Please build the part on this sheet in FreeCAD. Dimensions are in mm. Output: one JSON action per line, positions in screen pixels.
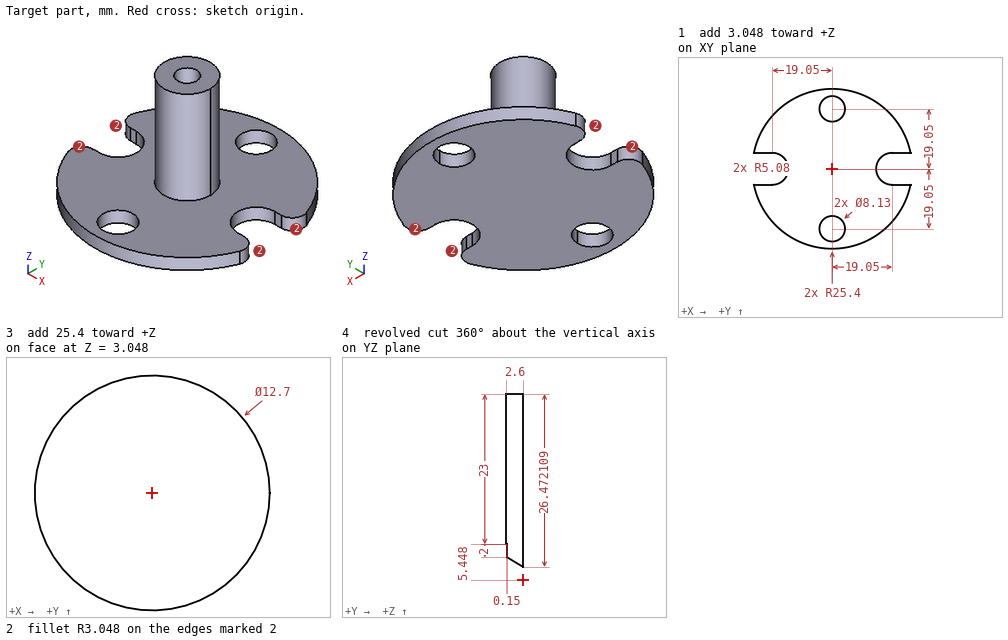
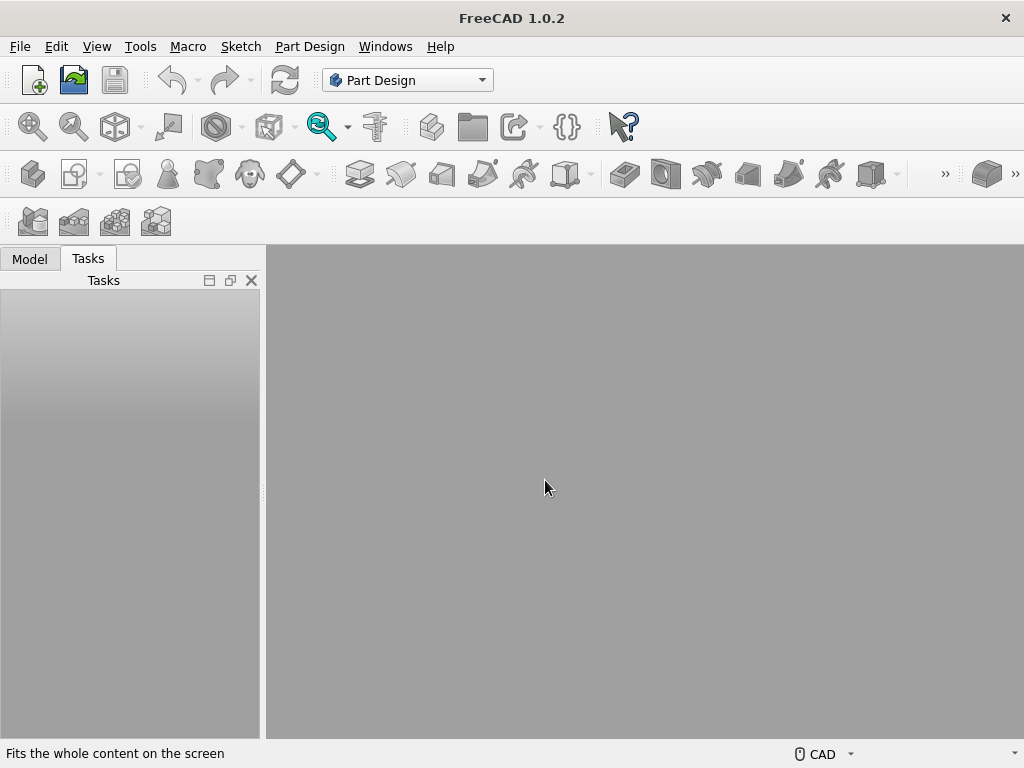
{"action": "left_click", "coordinate": [33, 80]}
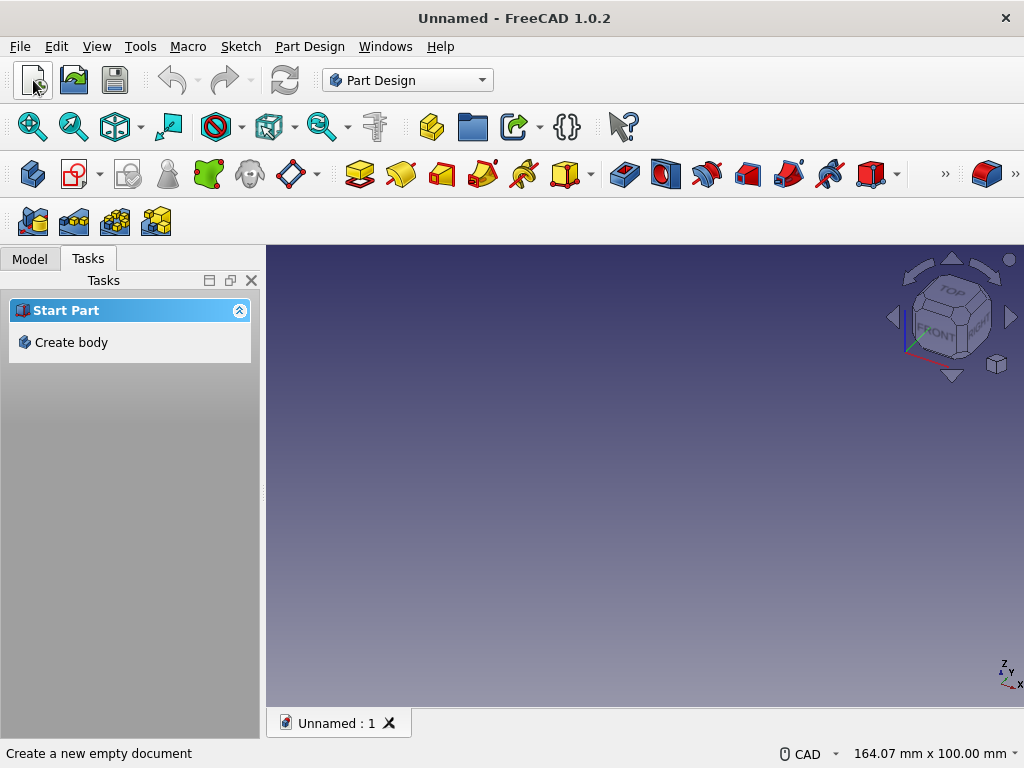
{"action": "left_click", "coordinate": [74, 174]}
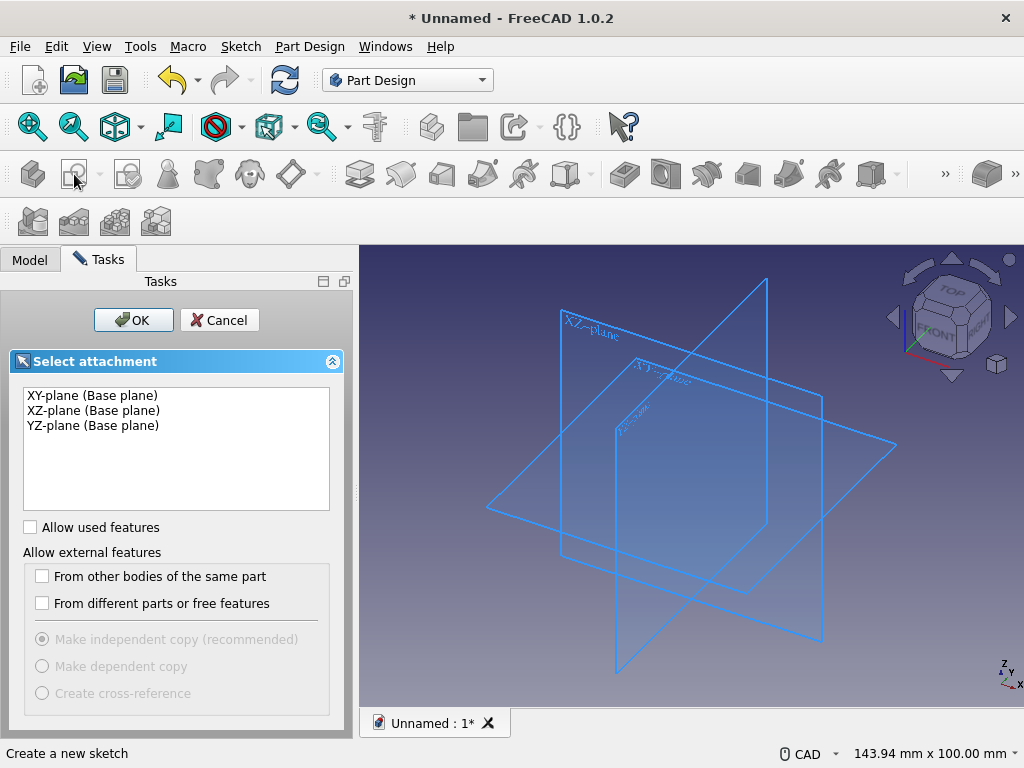
{"action": "left_click", "coordinate": [84, 396]}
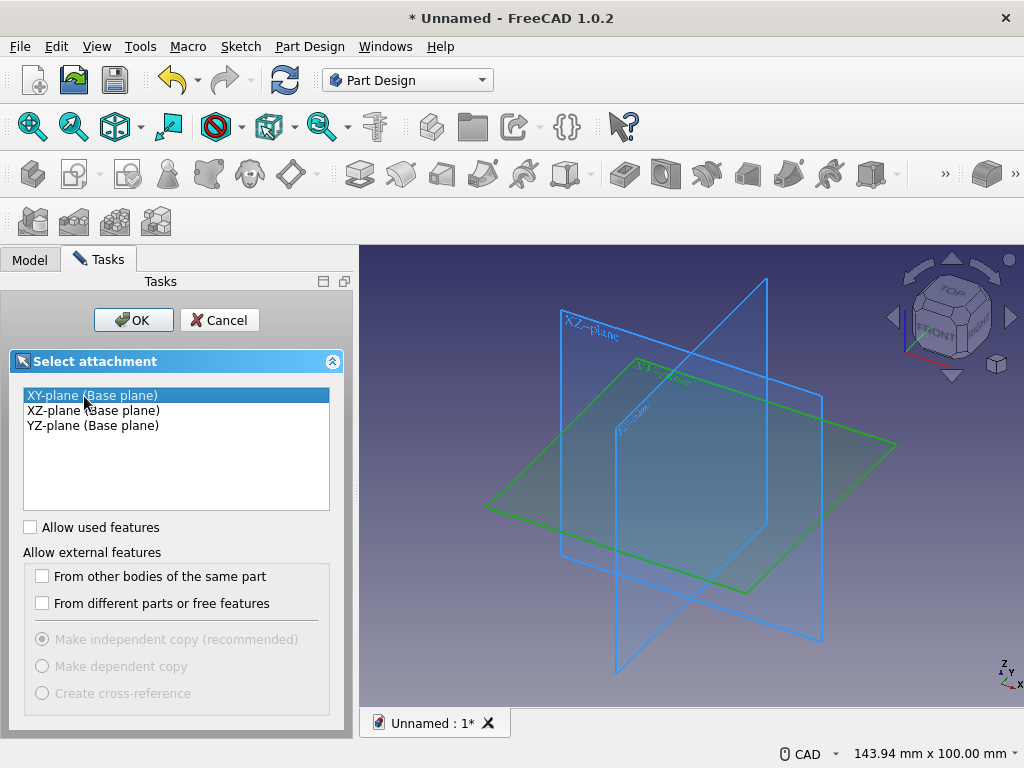
{"action": "left_click", "coordinate": [134, 320]}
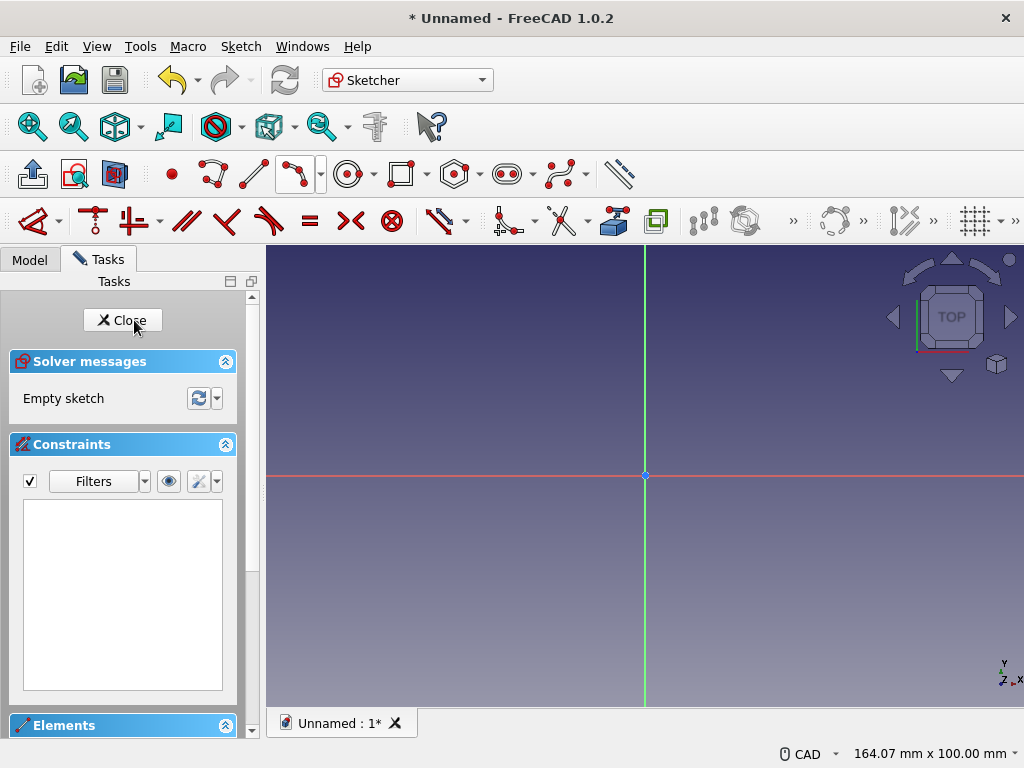
{"action": "left_click", "coordinate": [254, 174]}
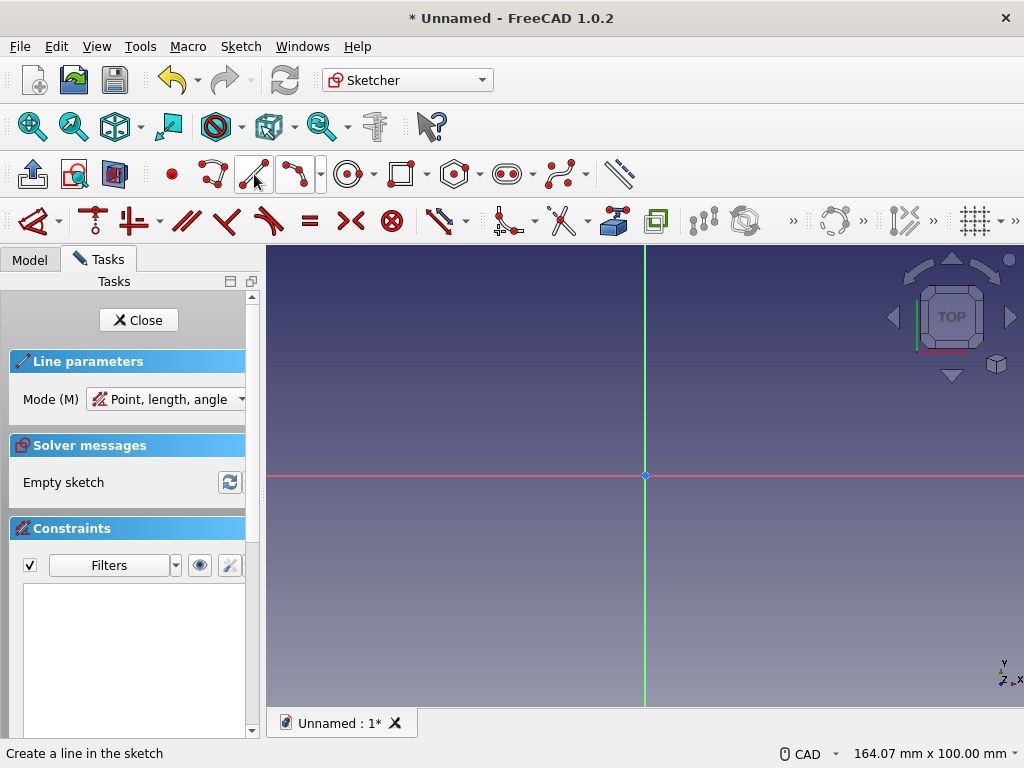
{"action": "left_click", "coordinate": [530, 453]}
{"action": "left_click", "coordinate": [557, 453]}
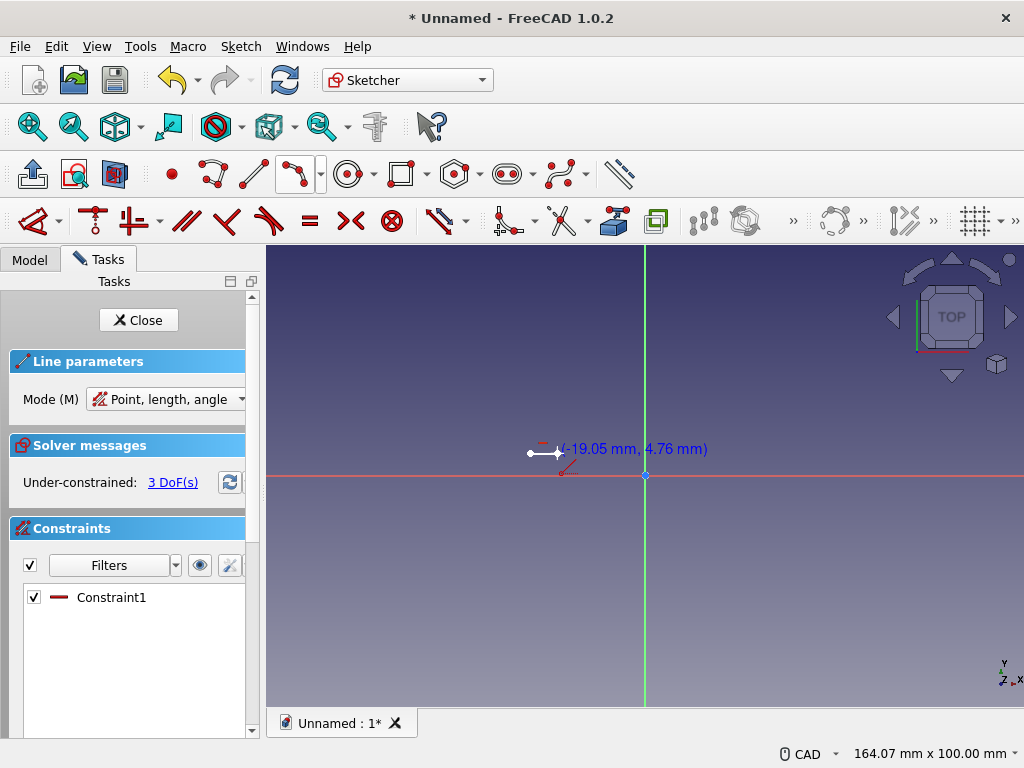
{"action": "left_click", "coordinate": [557, 499]}
{"action": "left_click", "coordinate": [530, 499]}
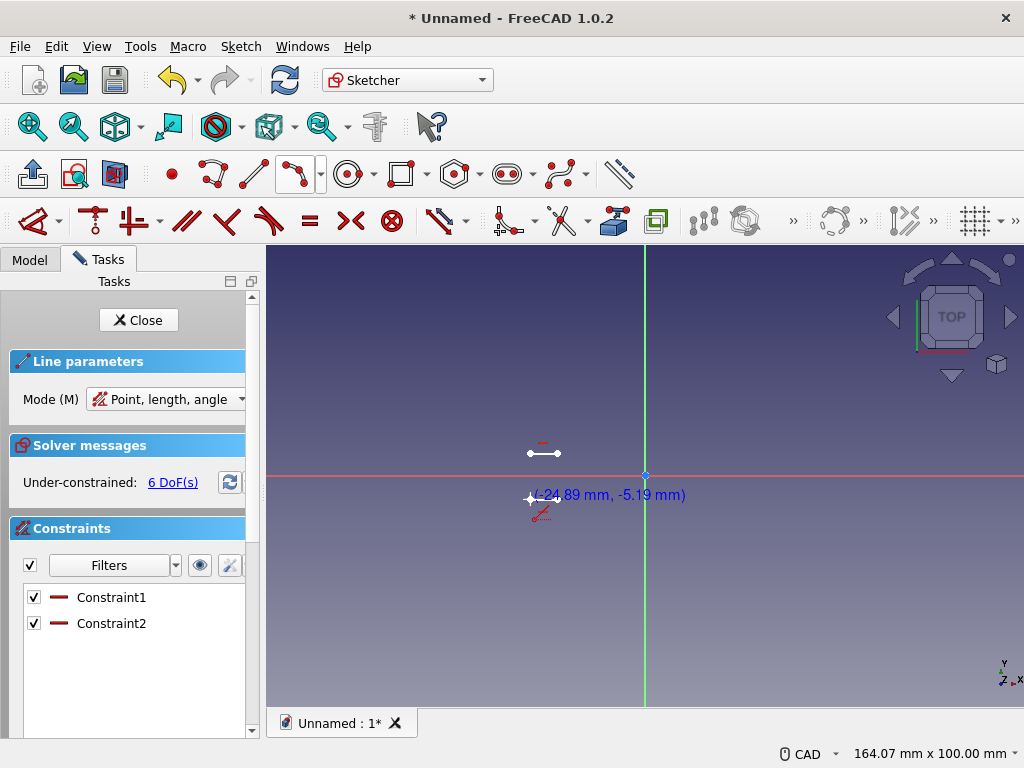
{"action": "left_click", "coordinate": [760, 499]}
{"action": "left_click", "coordinate": [733, 499]}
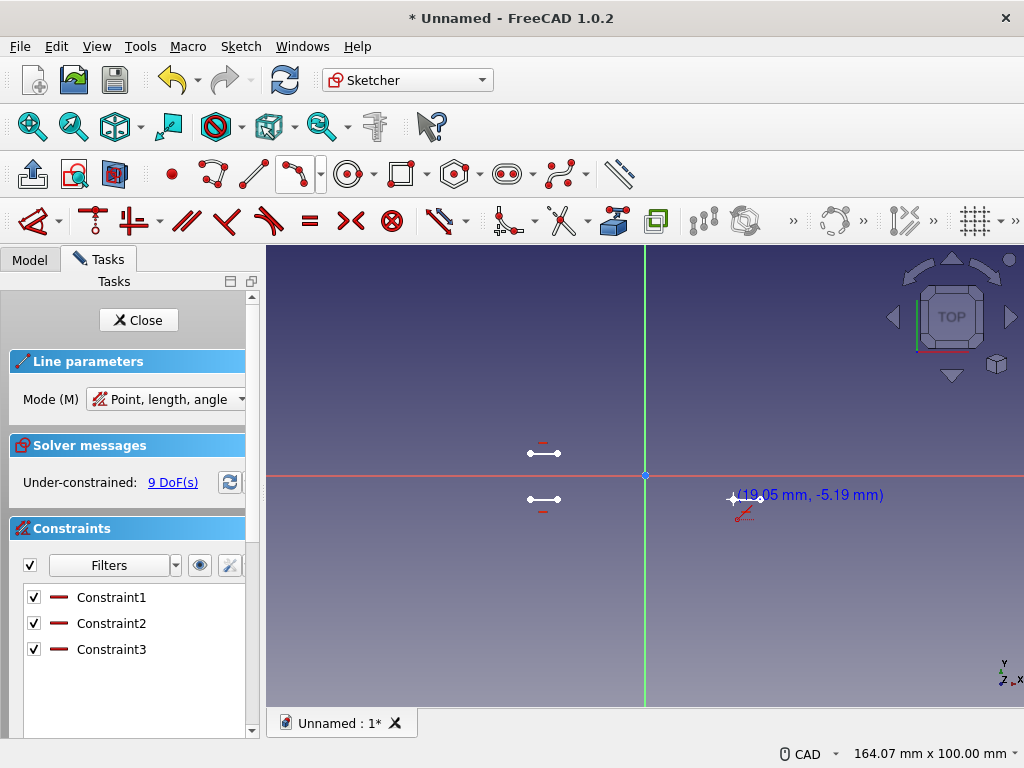
{"action": "left_click", "coordinate": [733, 453]}
{"action": "left_click", "coordinate": [760, 453]}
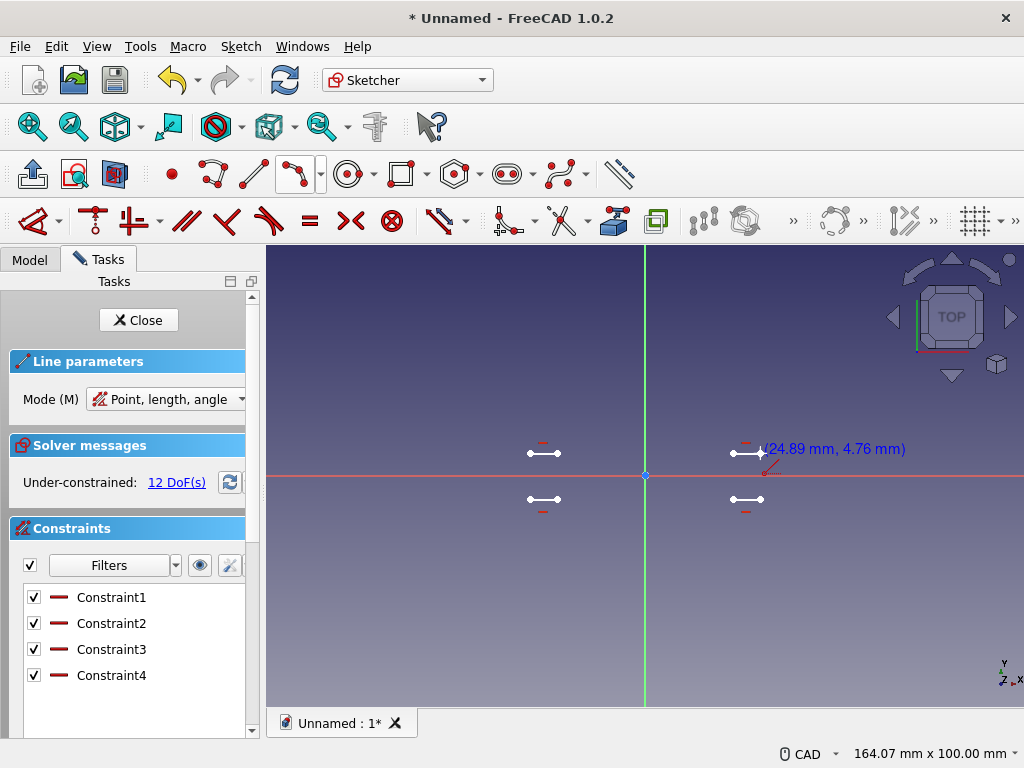
{"action": "left_click", "coordinate": [294, 174]}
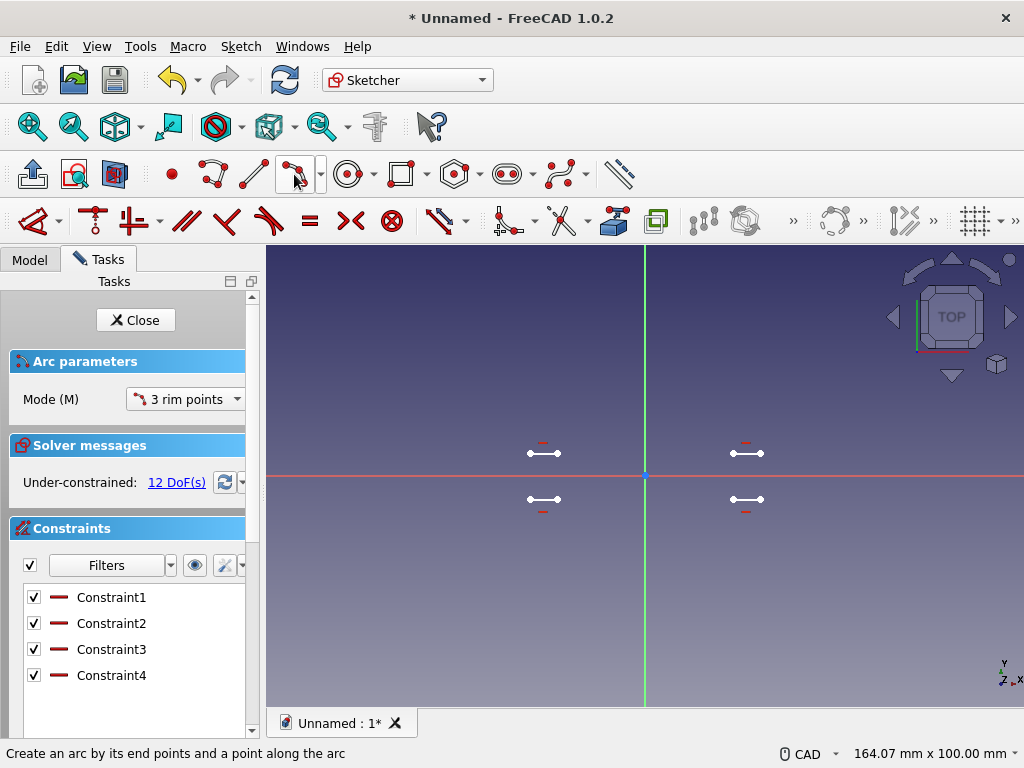
{"action": "left_click", "coordinate": [557, 454]}
{"action": "left_click", "coordinate": [557, 500]}
{"action": "left_click", "coordinate": [576, 490]}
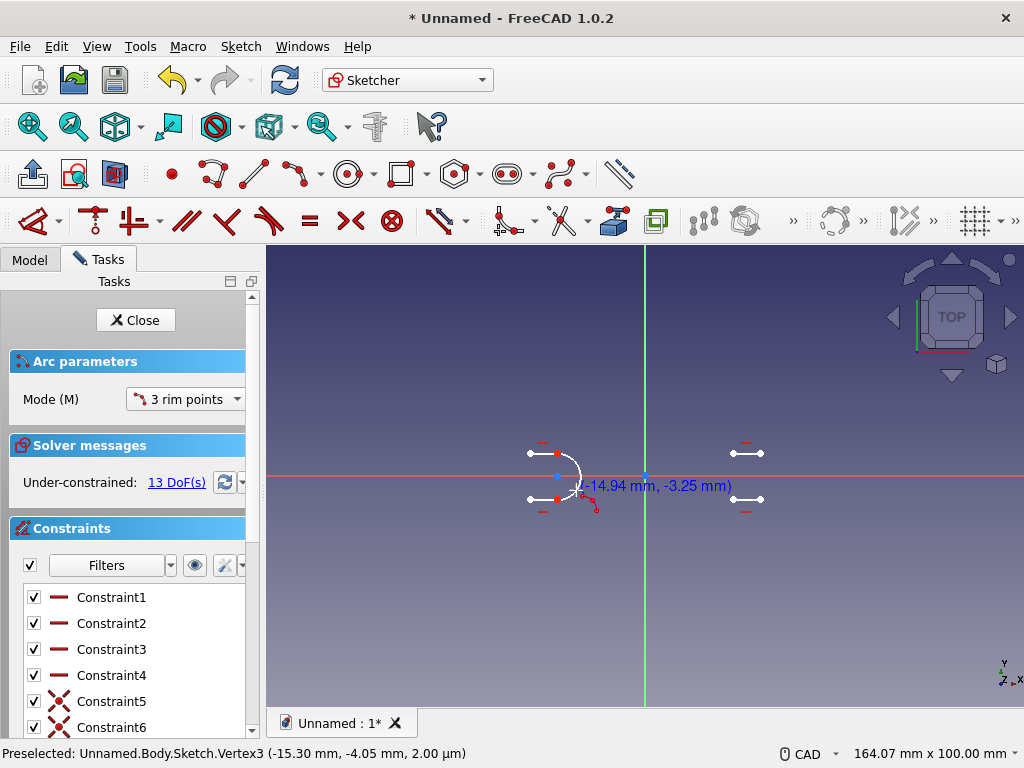
{"action": "left_click", "coordinate": [530, 500]}
{"action": "left_click", "coordinate": [760, 500]}
{"action": "left_click", "coordinate": [613, 589]}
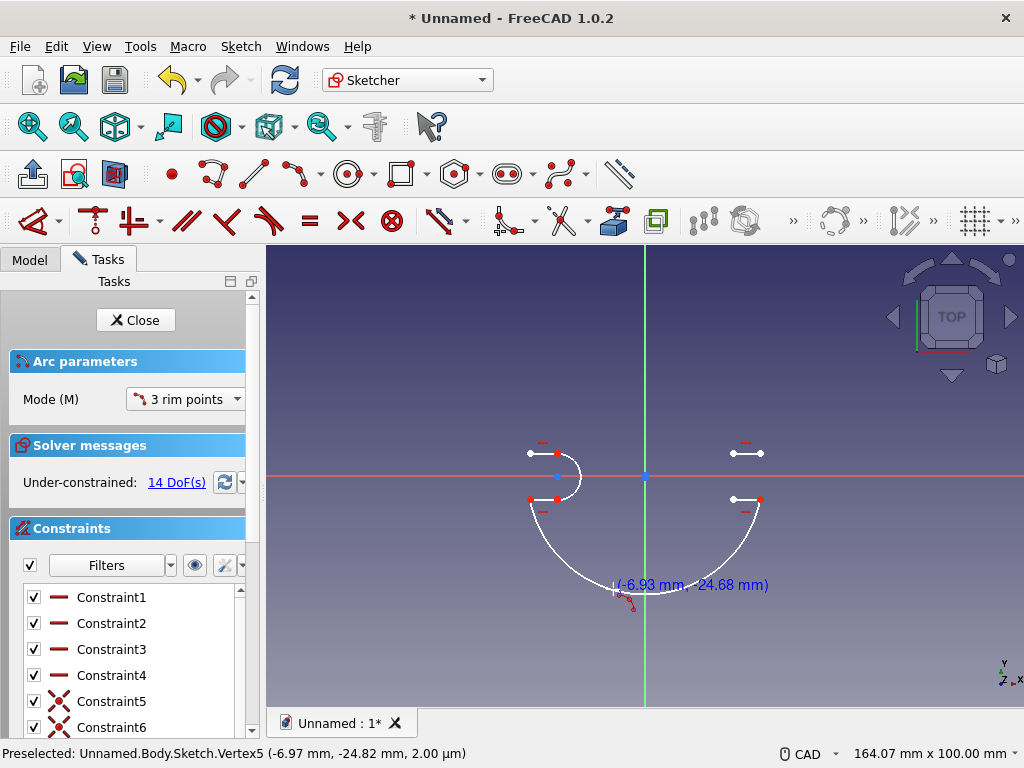
{"action": "left_click", "coordinate": [733, 500]}
{"action": "left_click", "coordinate": [733, 454]}
{"action": "left_click", "coordinate": [714, 462]}